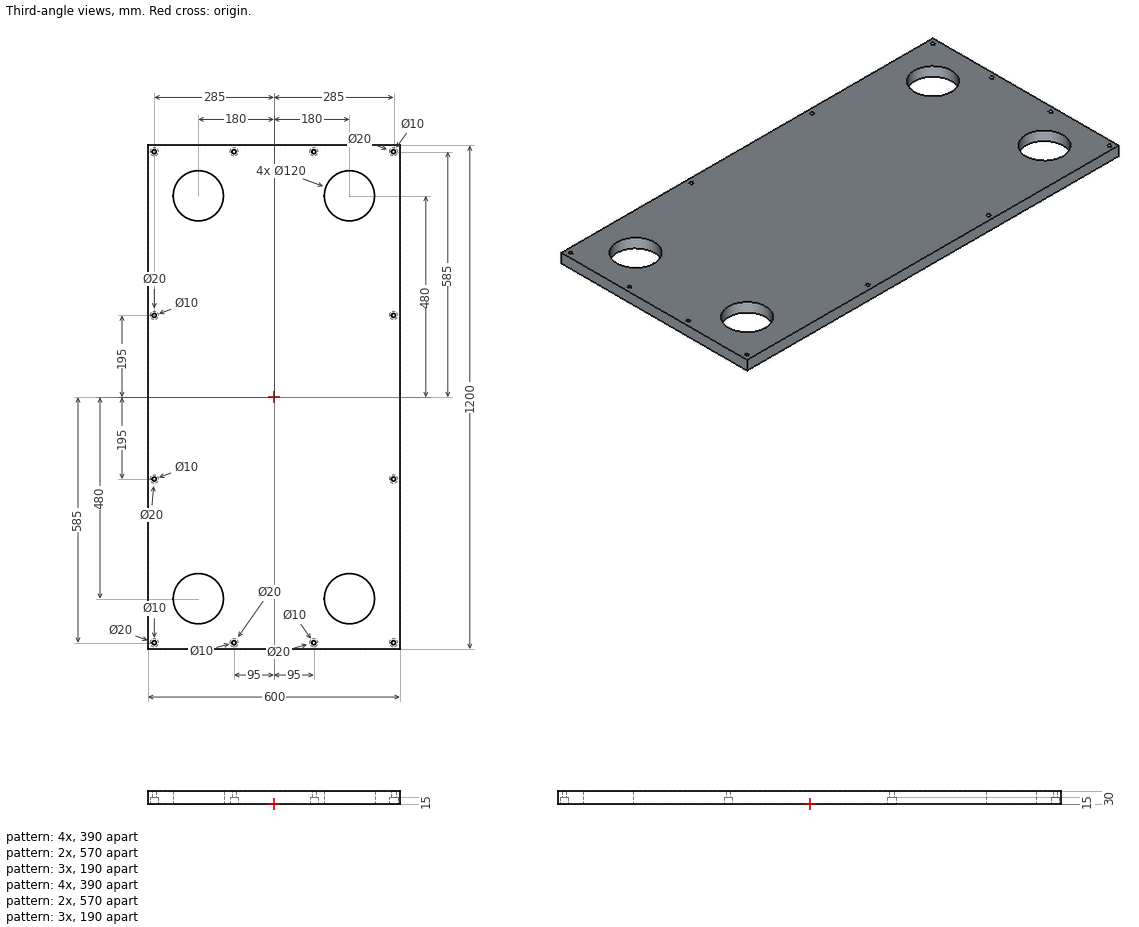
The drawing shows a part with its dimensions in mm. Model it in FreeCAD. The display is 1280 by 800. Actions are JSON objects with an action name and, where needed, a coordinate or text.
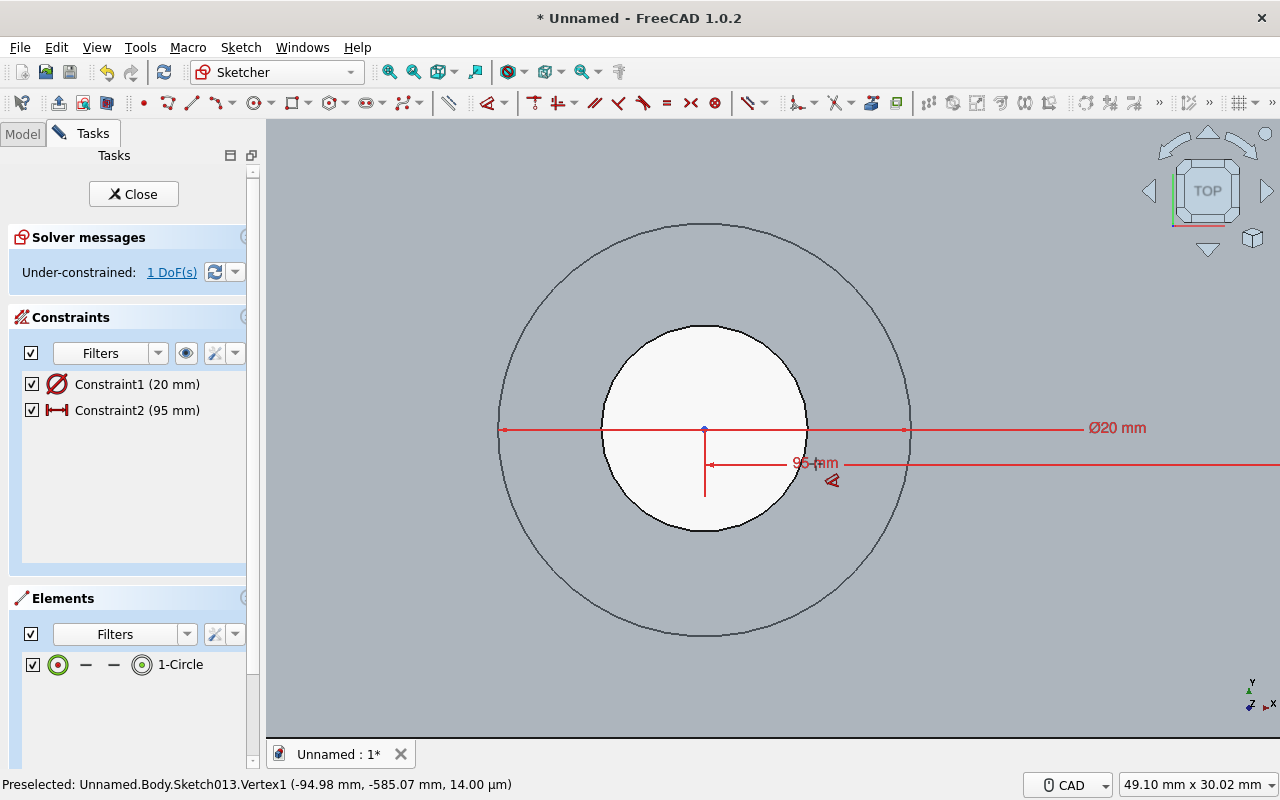
{"action": "left_click", "coordinate": [705, 430]}
{"action": "left_click", "coordinate": [671, 288]}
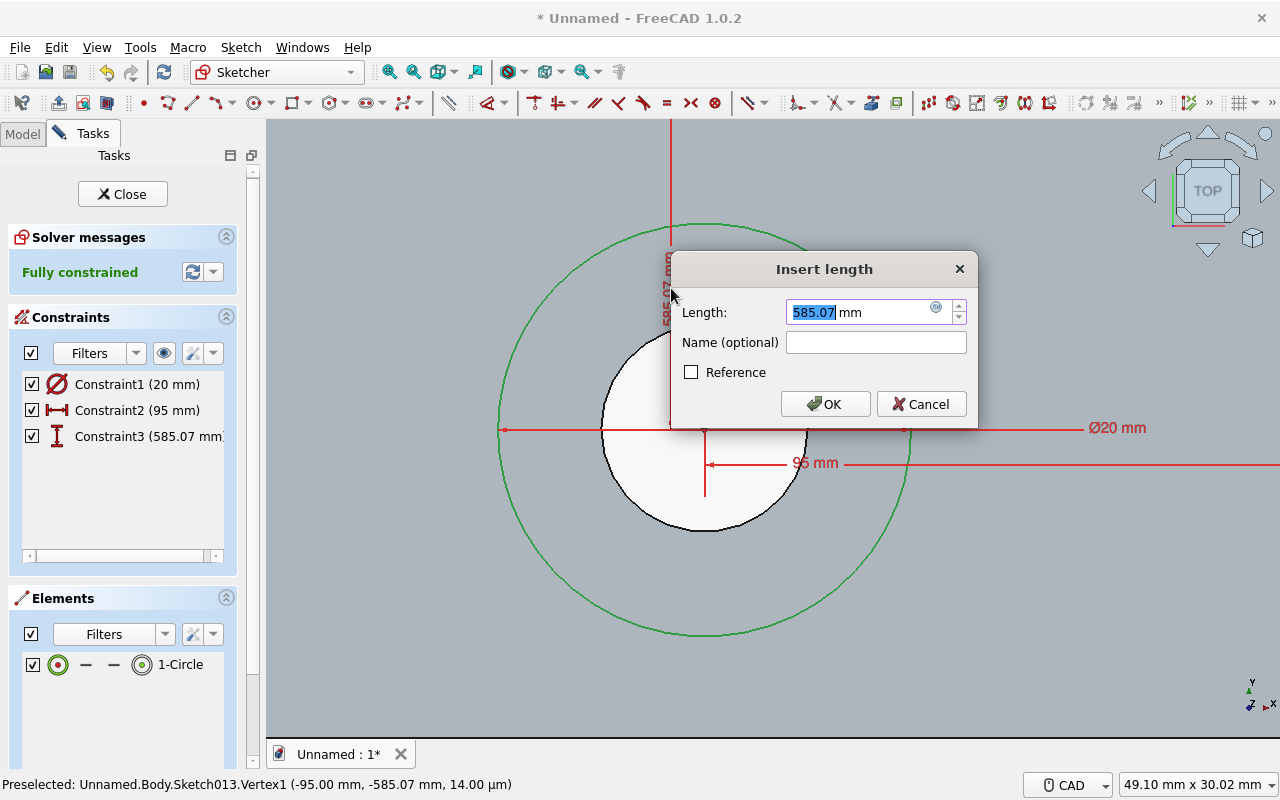
{"action": "type", "text": "585"}
{"action": "key", "text": "Return"}
{"action": "key", "text": "Escape"}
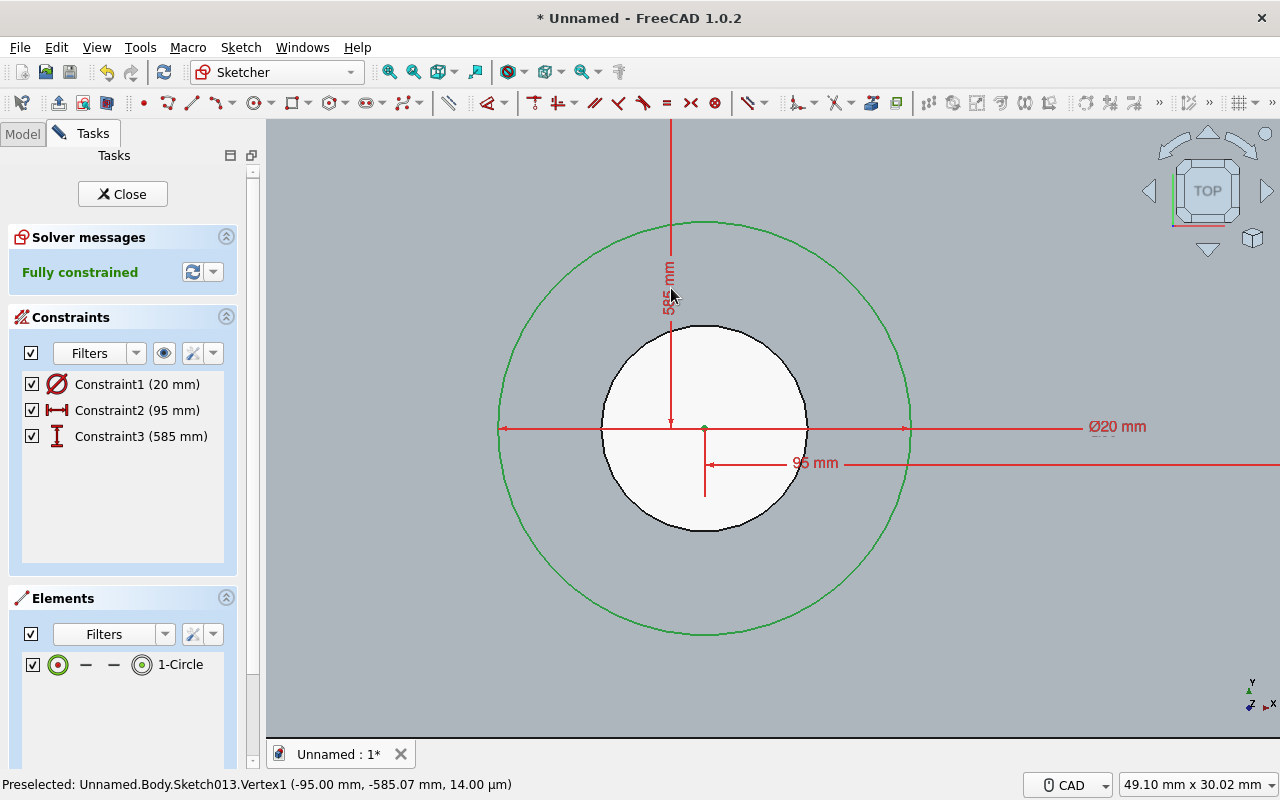
{"action": "left_click", "coordinate": [123, 194]}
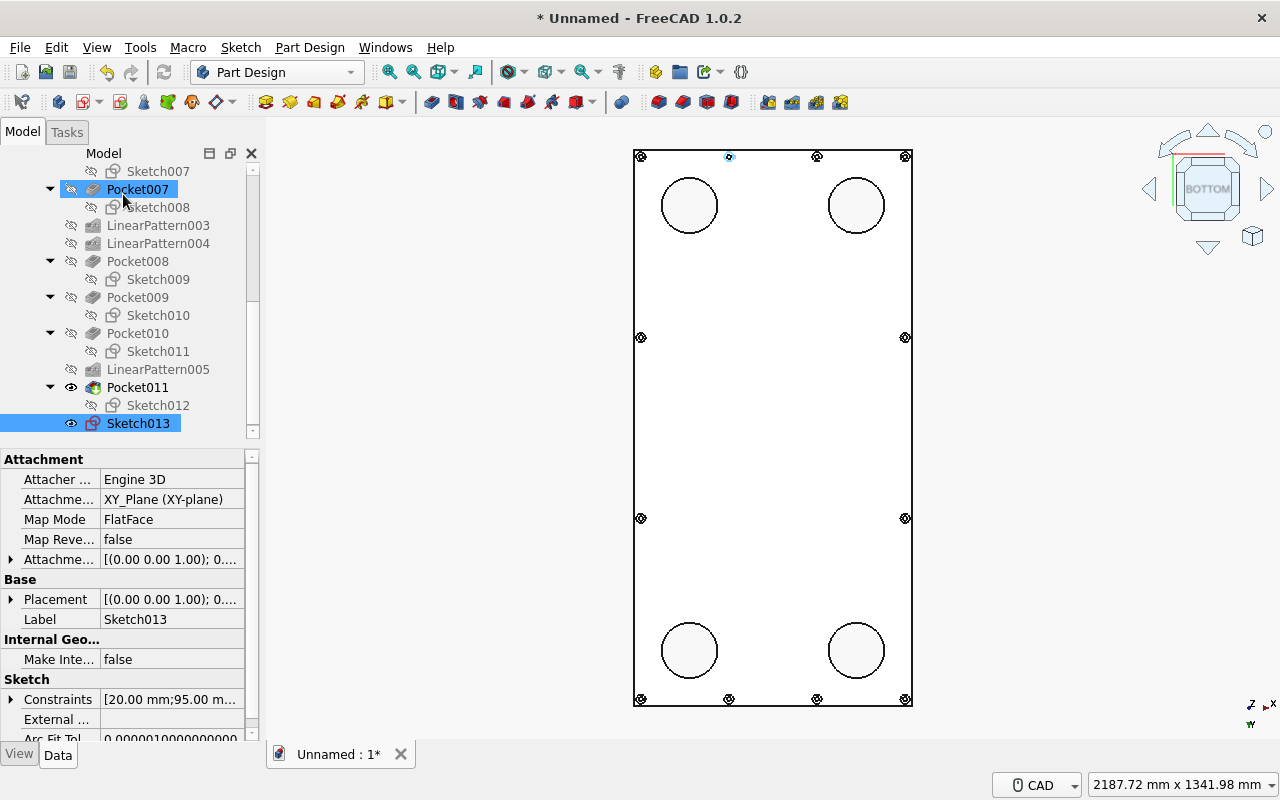
{"action": "left_click", "coordinate": [432, 102]}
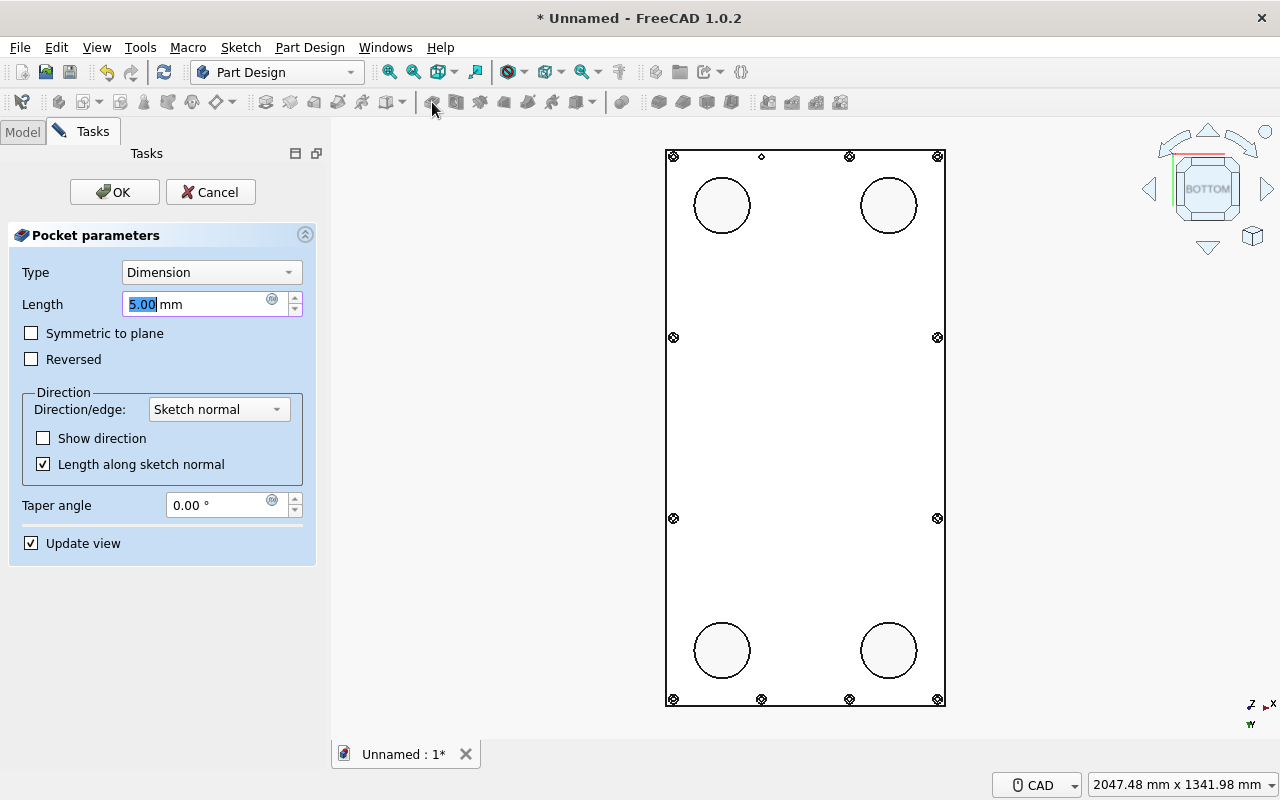
{"action": "type", "text": "15"}
{"action": "key", "text": "Tab"}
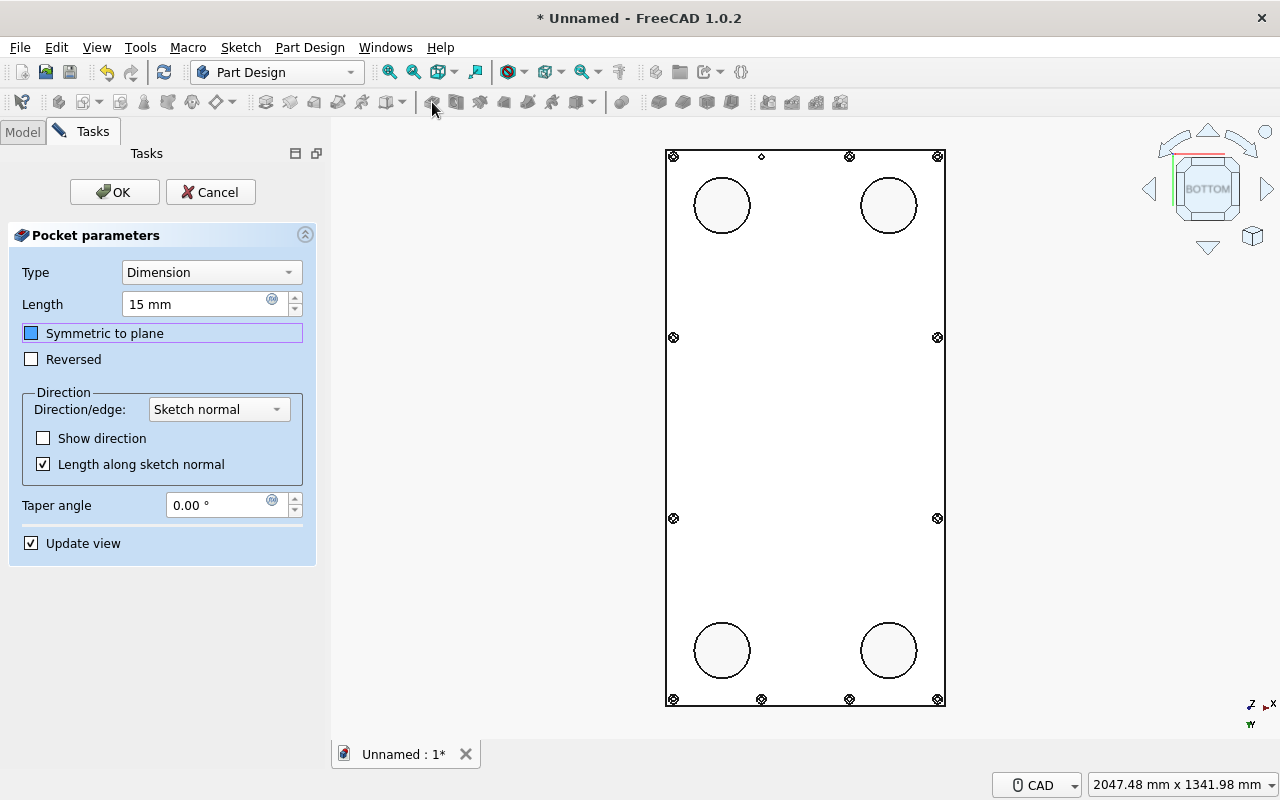
{"action": "left_click", "coordinate": [30, 359]}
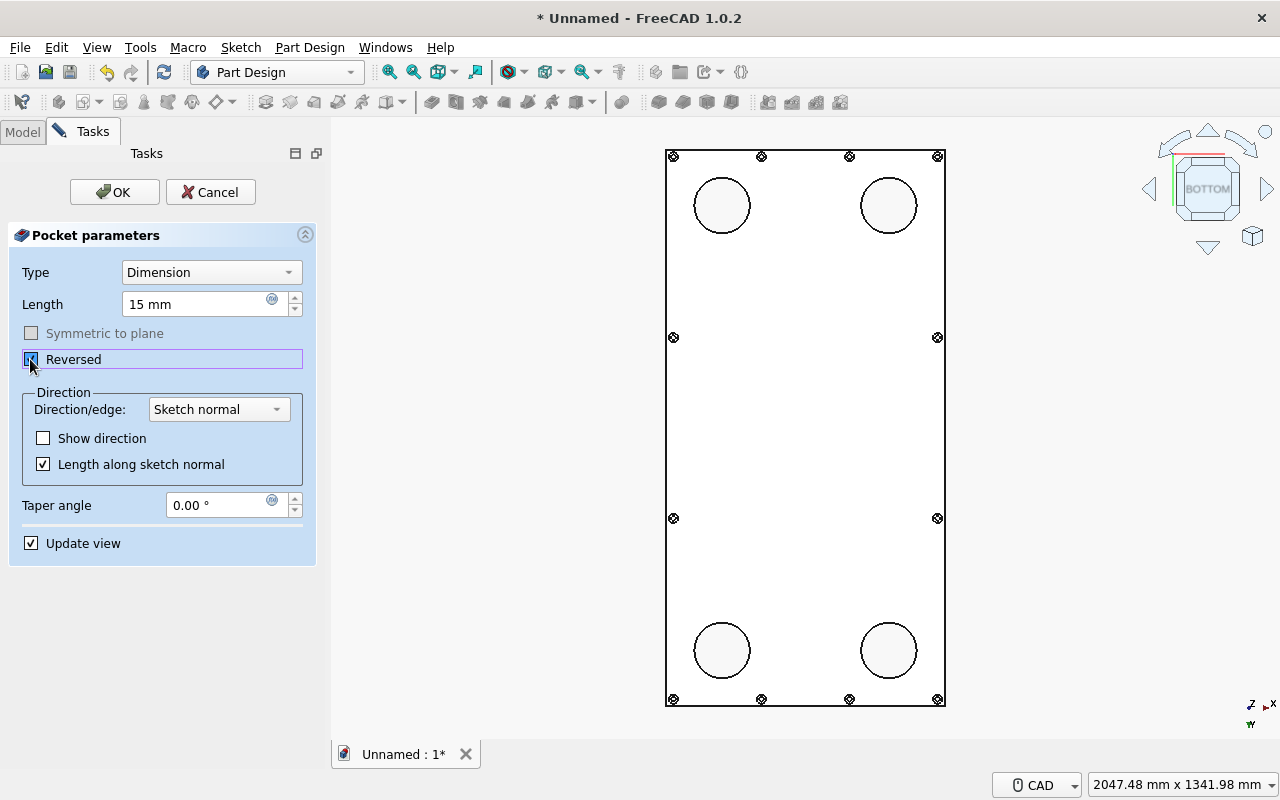
{"action": "left_click", "coordinate": [115, 192]}